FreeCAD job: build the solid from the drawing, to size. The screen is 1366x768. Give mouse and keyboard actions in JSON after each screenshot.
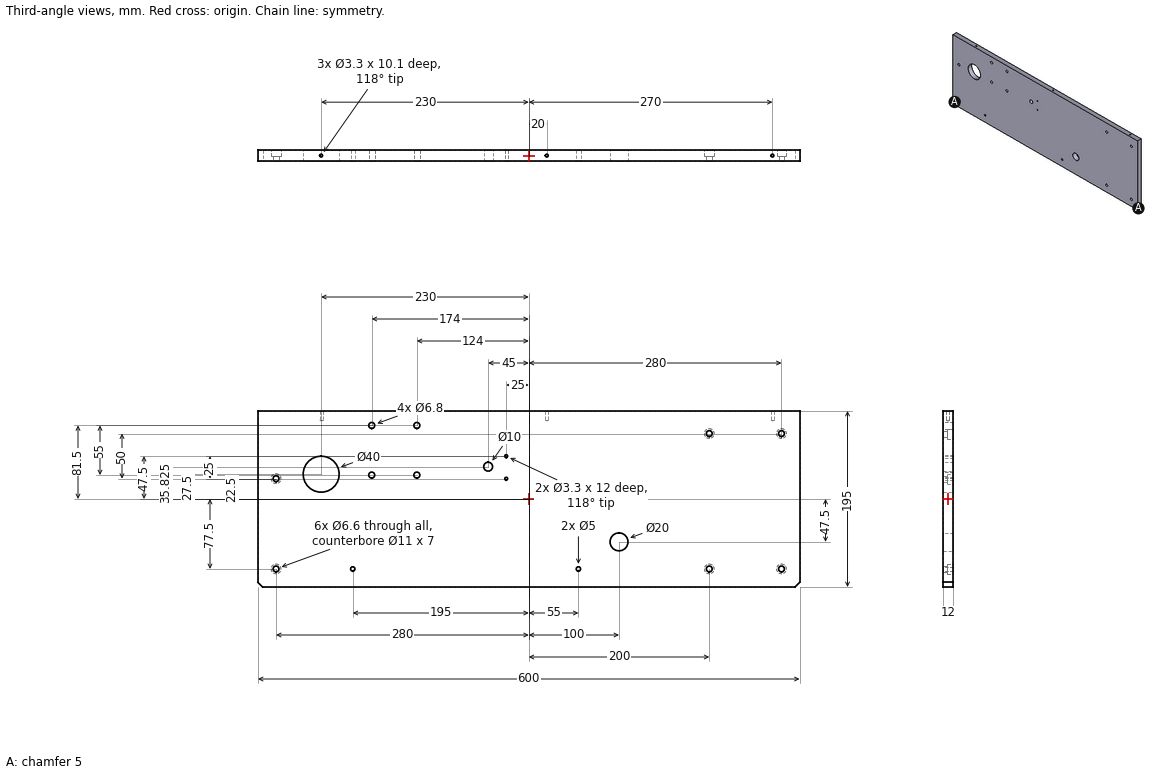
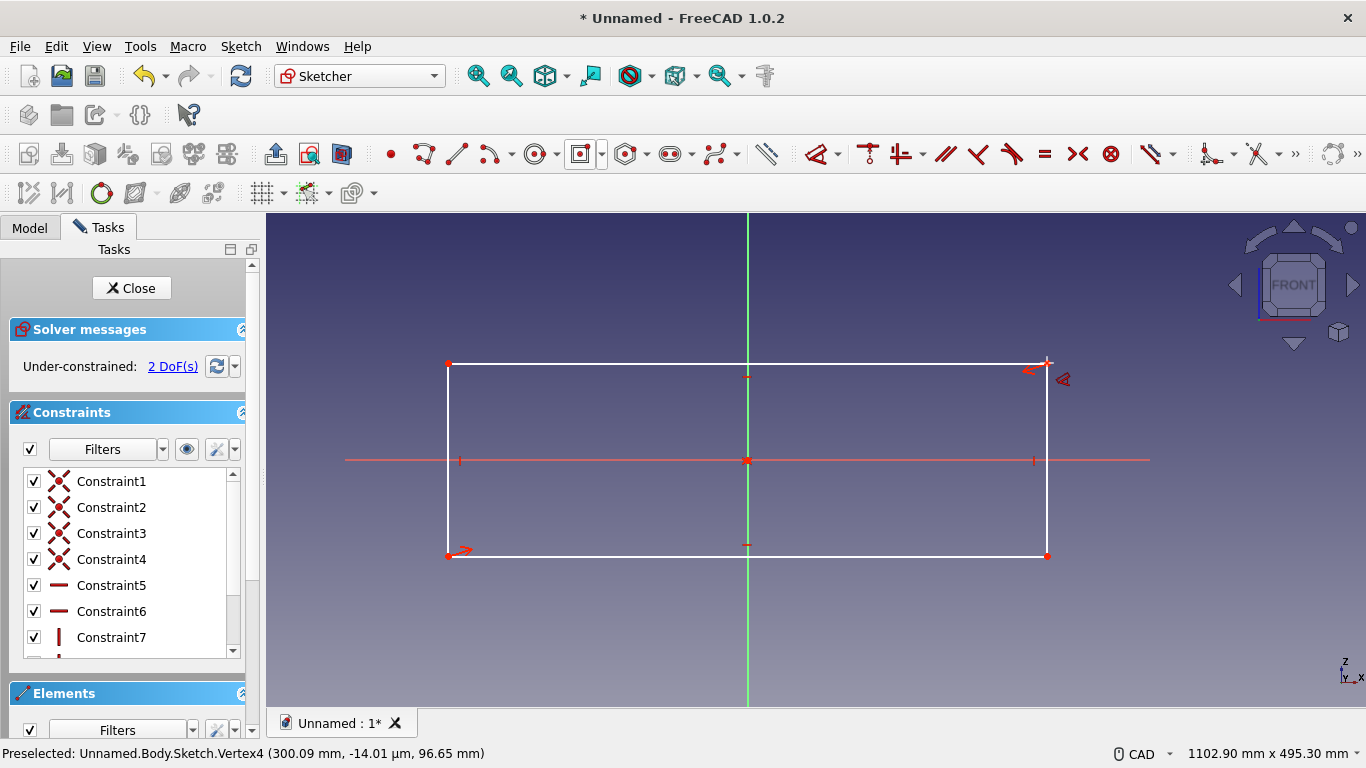
{"action": "left_click", "coordinate": [628, 557]}
{"action": "left_click", "coordinate": [610, 591]}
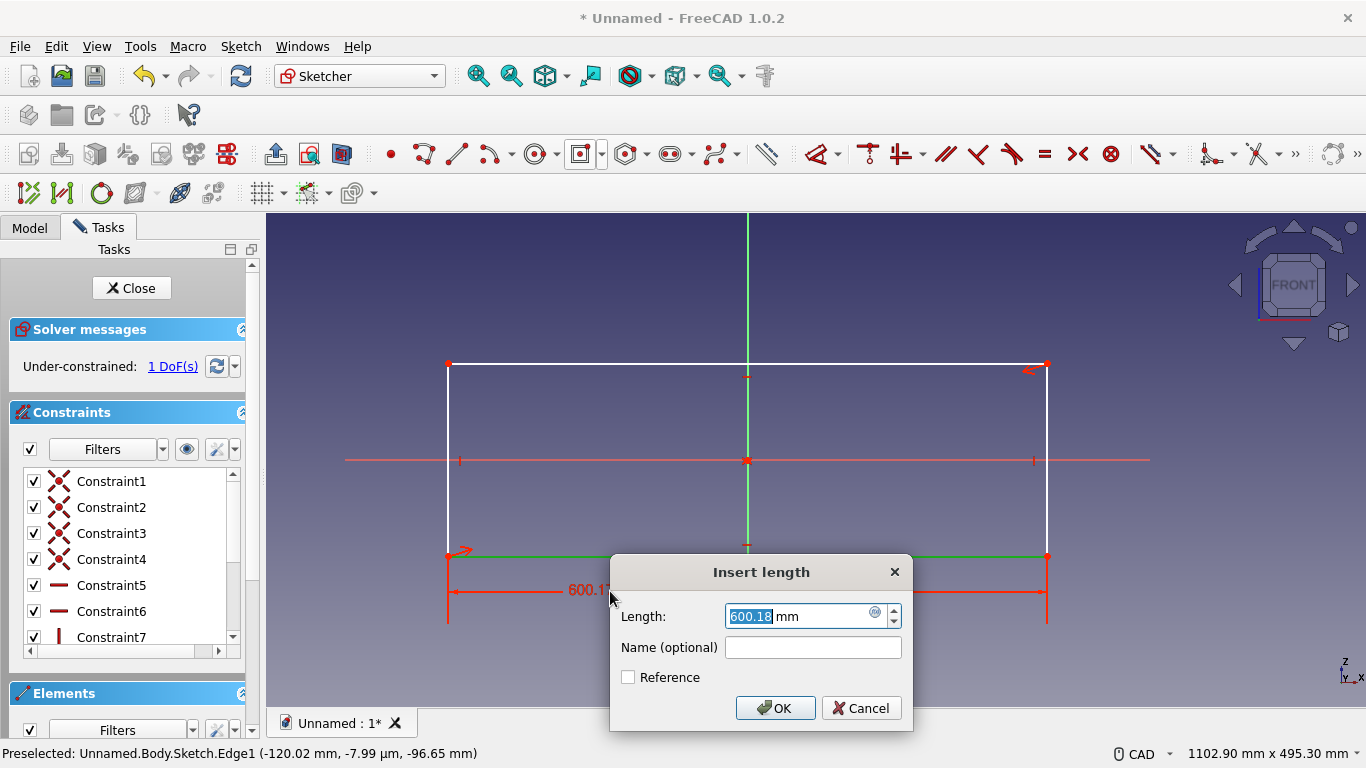
{"action": "type", "text": "600"}
{"action": "key", "text": "Return"}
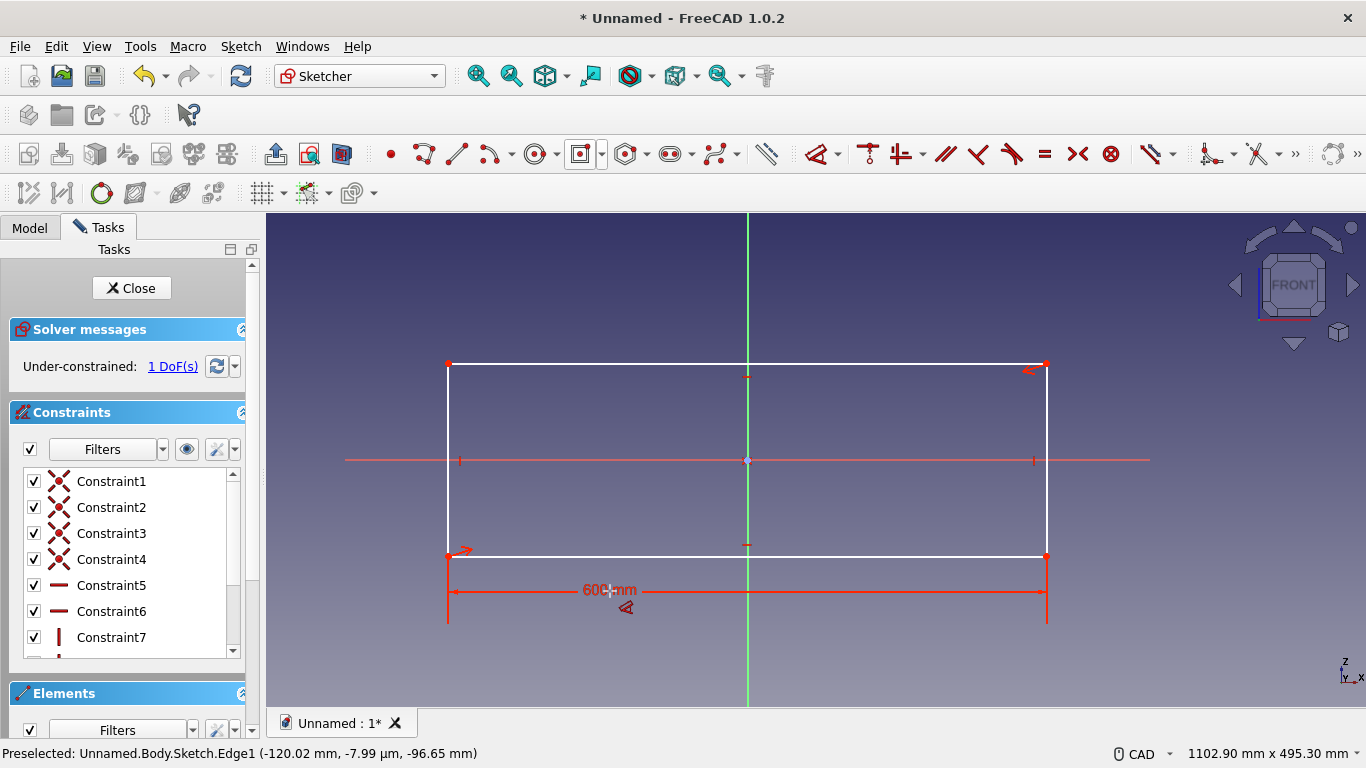
{"action": "left_click", "coordinate": [1047, 499]}
{"action": "left_click", "coordinate": [1081, 416]}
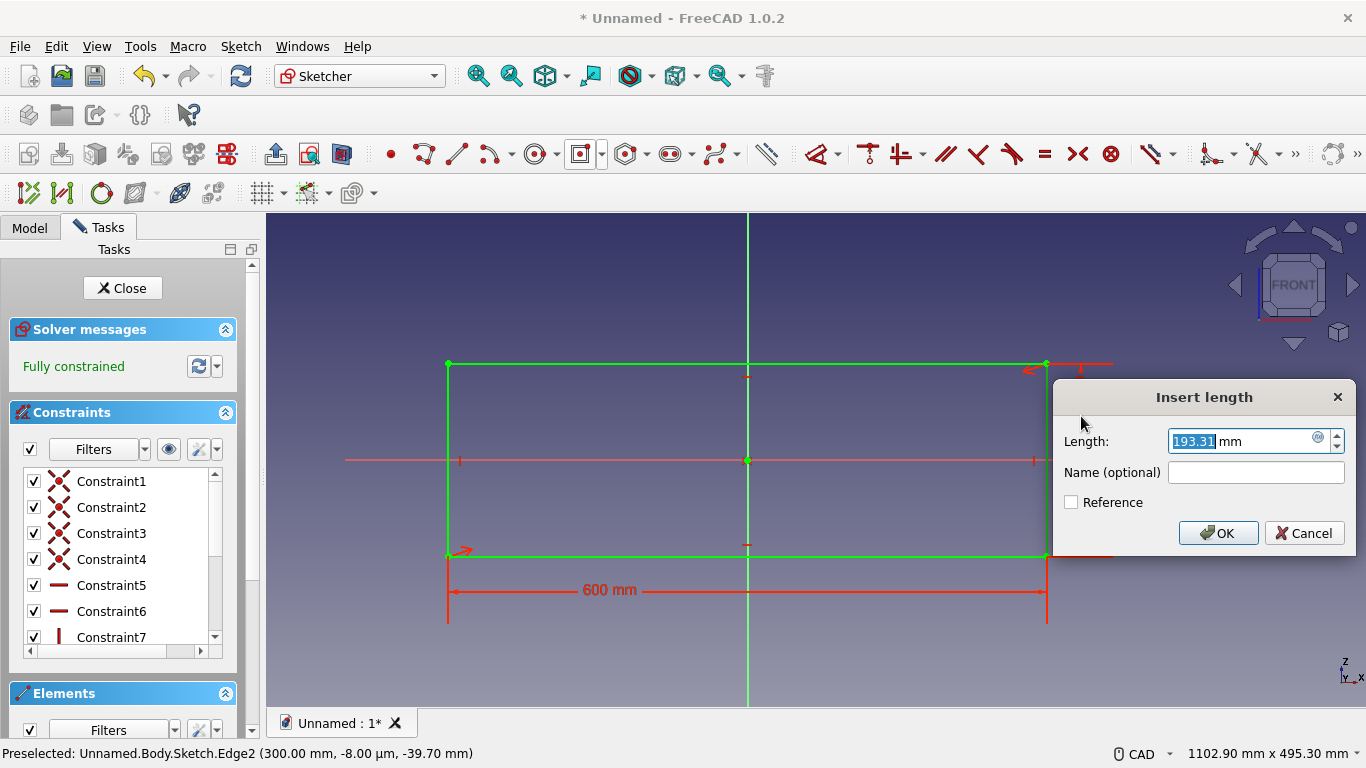
{"action": "type", "text": "195"}
{"action": "key", "text": "Return"}
{"action": "key", "text": "Escape"}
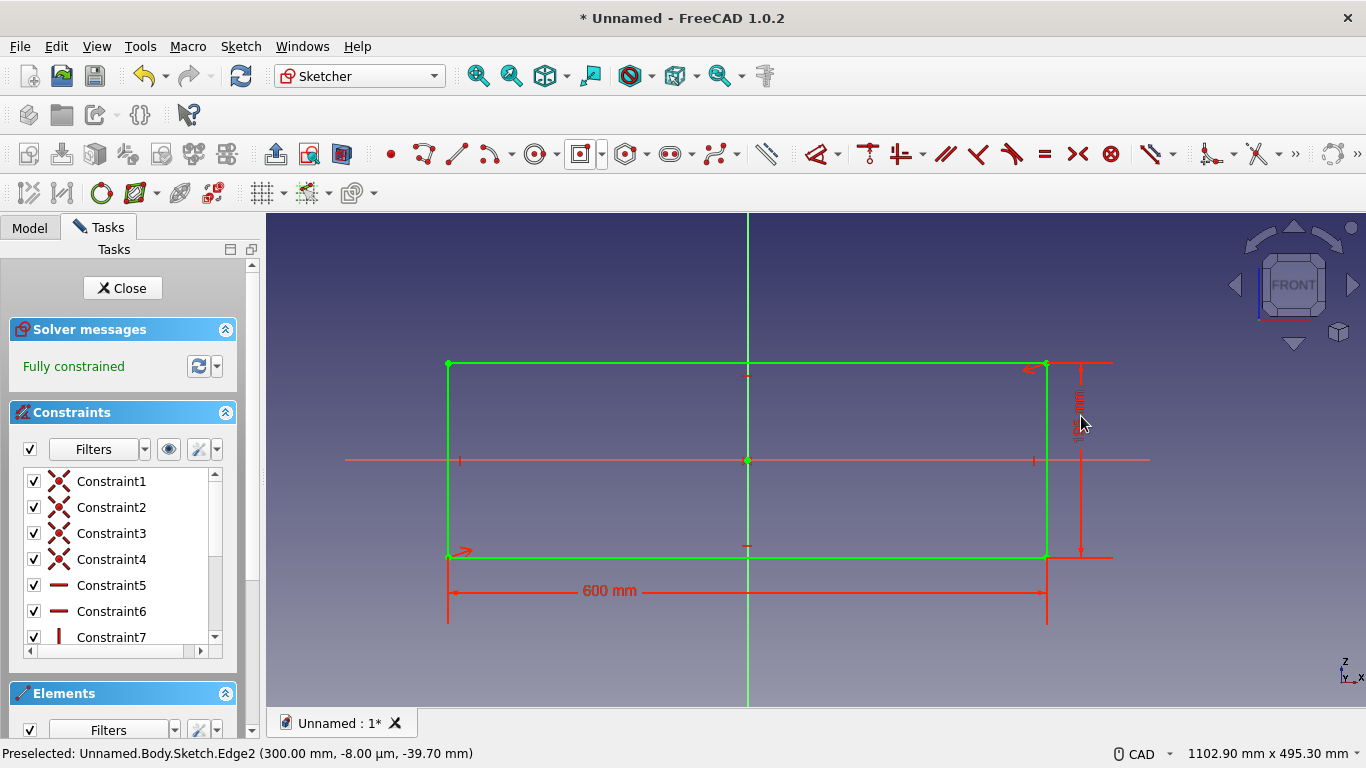
{"action": "left_click", "coordinate": [123, 288]}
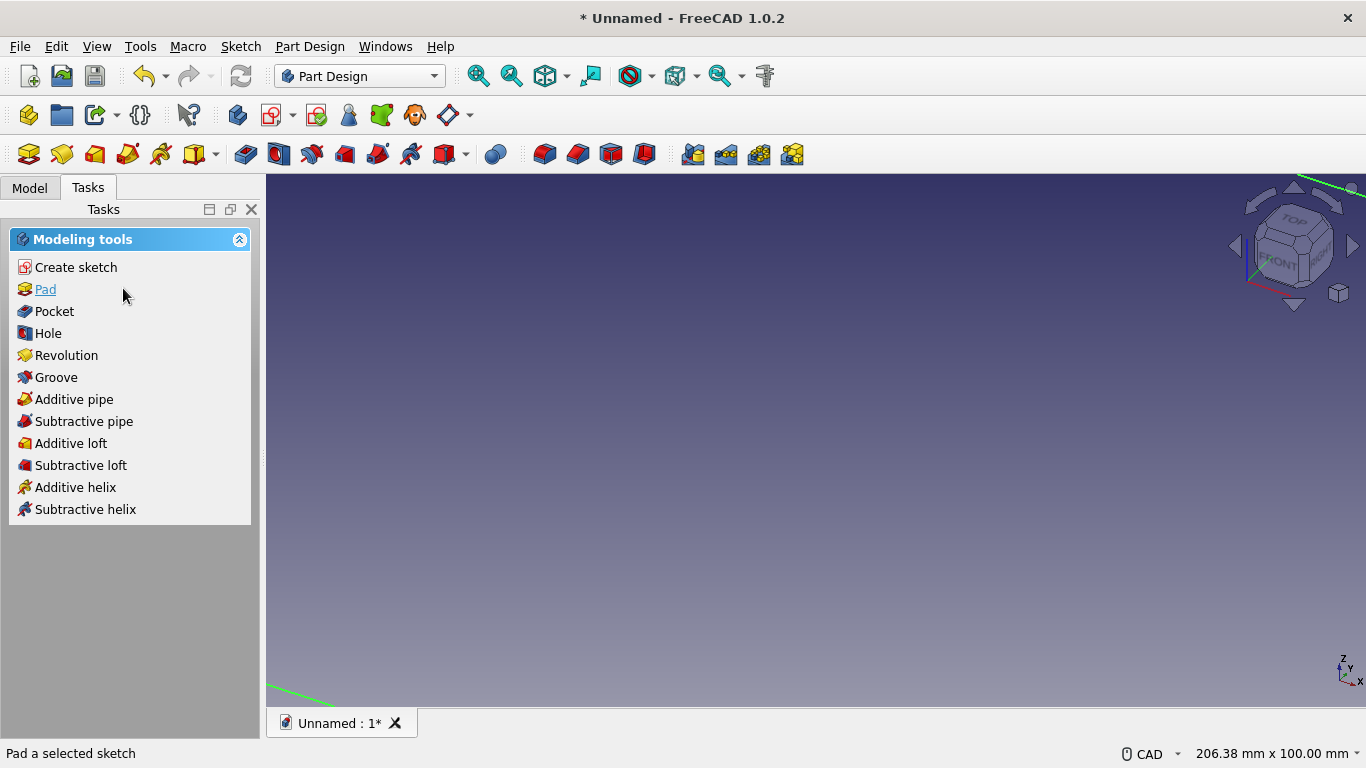
{"action": "left_click", "coordinate": [29, 154]}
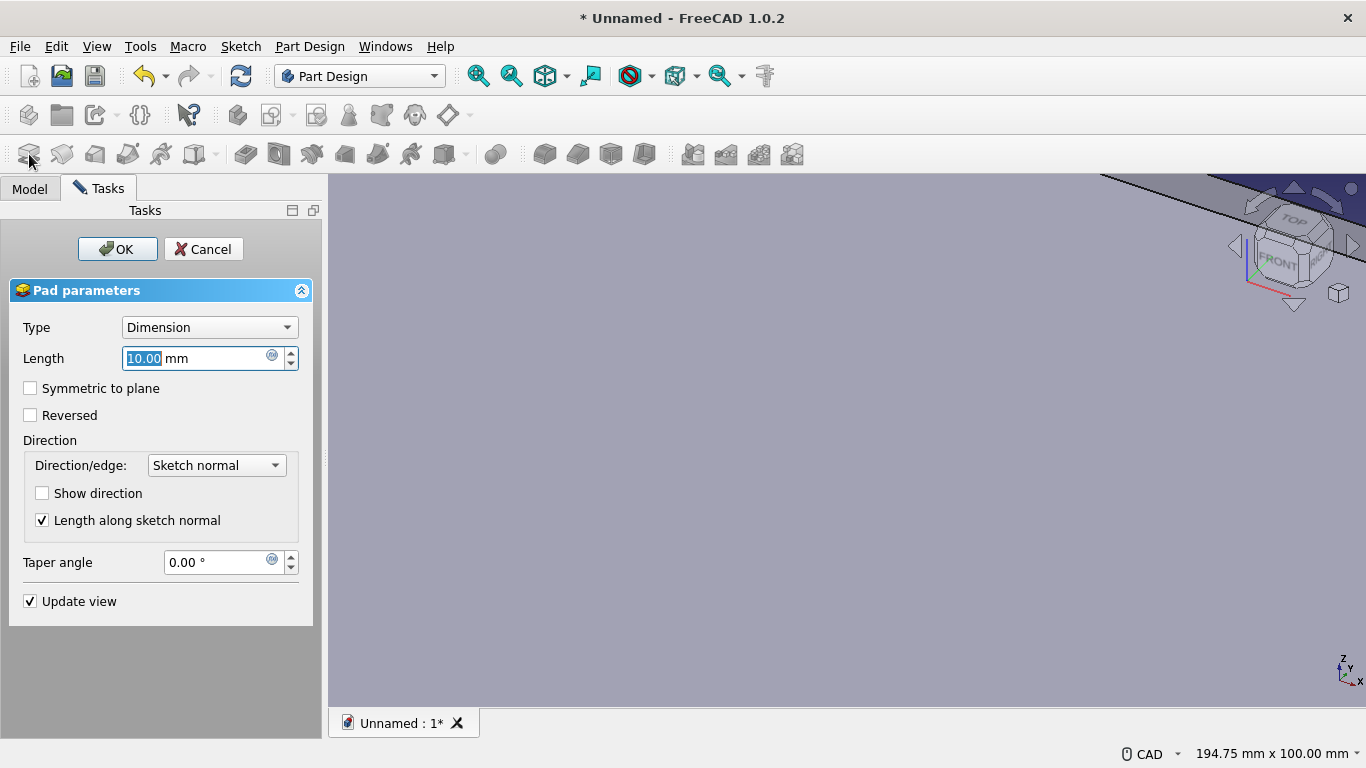
{"action": "type", "text": "12"}
{"action": "key", "text": "Tab"}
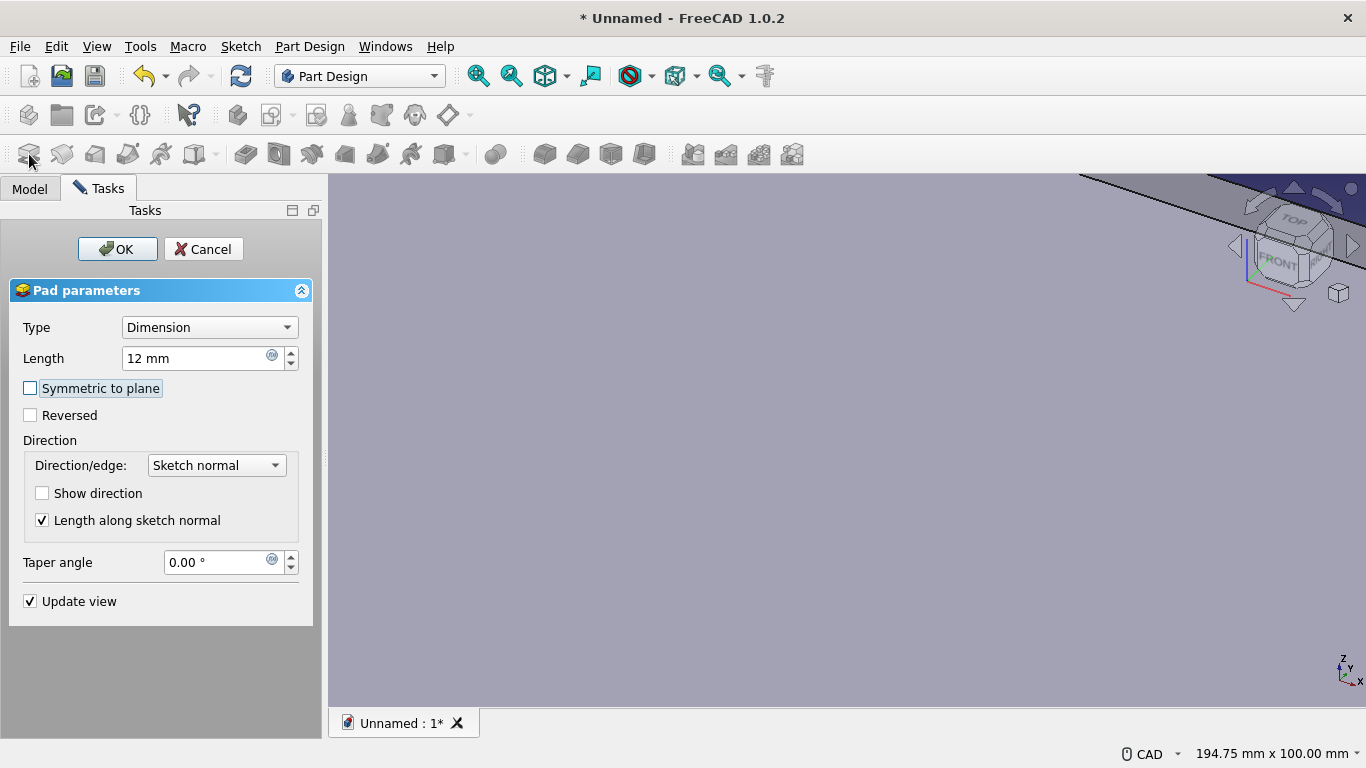
{"action": "left_click", "coordinate": [31, 388]}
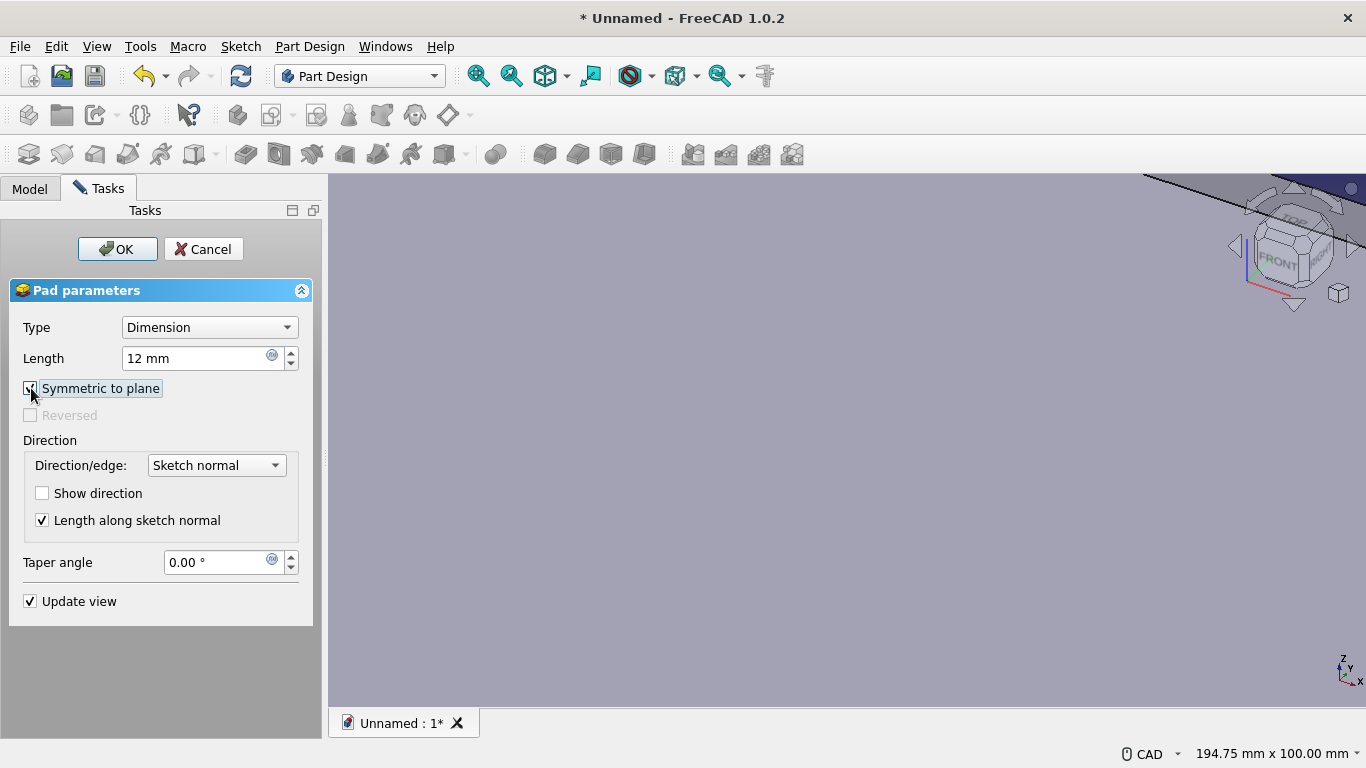
{"action": "left_click", "coordinate": [118, 249]}